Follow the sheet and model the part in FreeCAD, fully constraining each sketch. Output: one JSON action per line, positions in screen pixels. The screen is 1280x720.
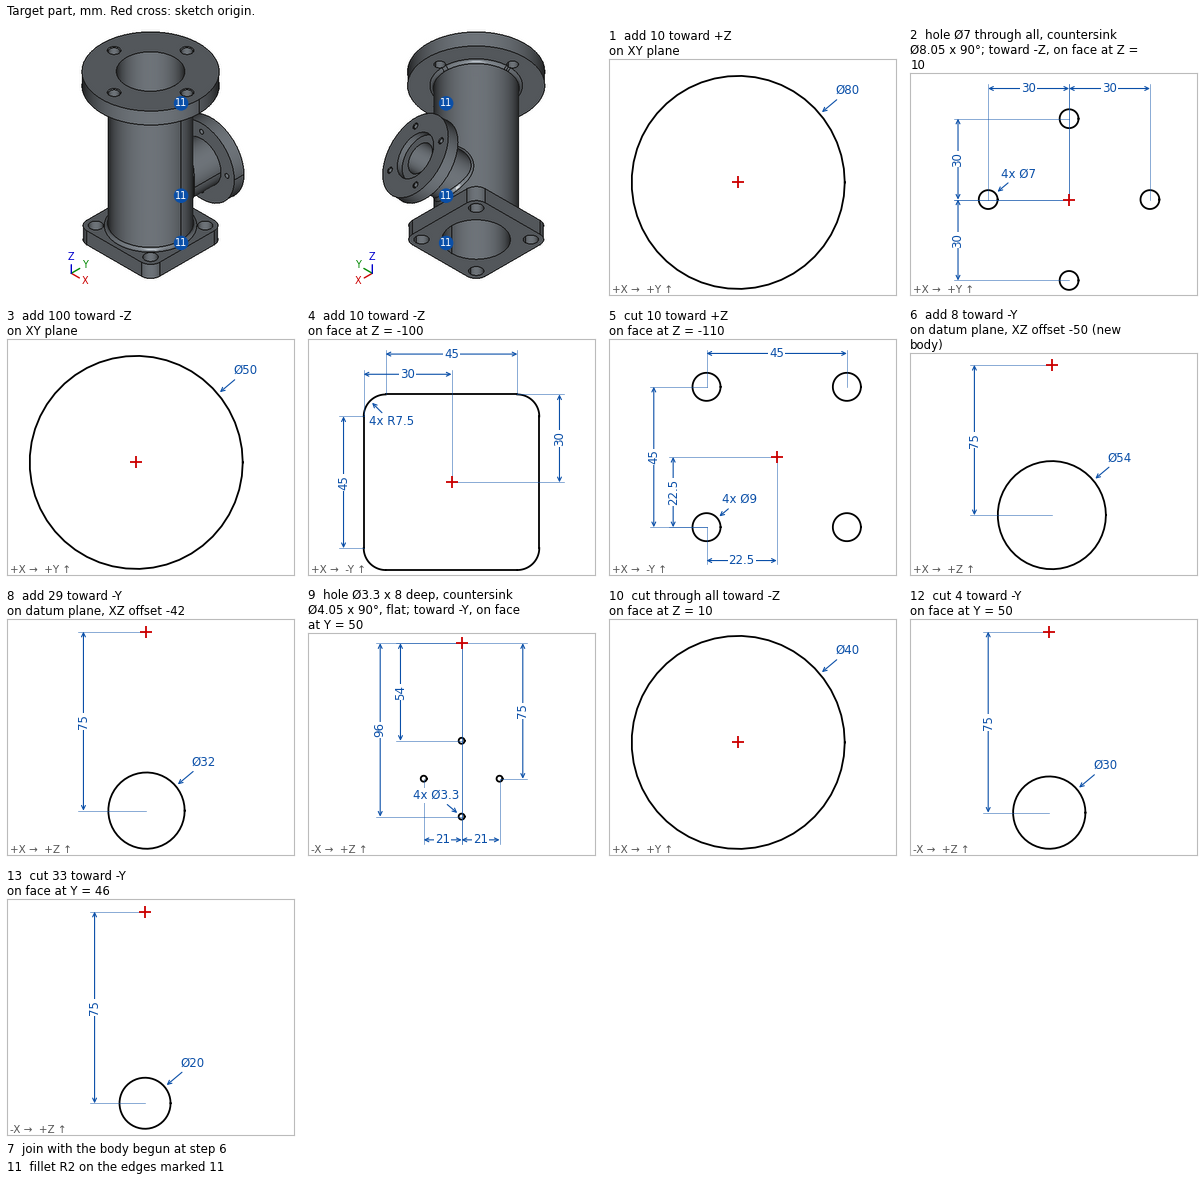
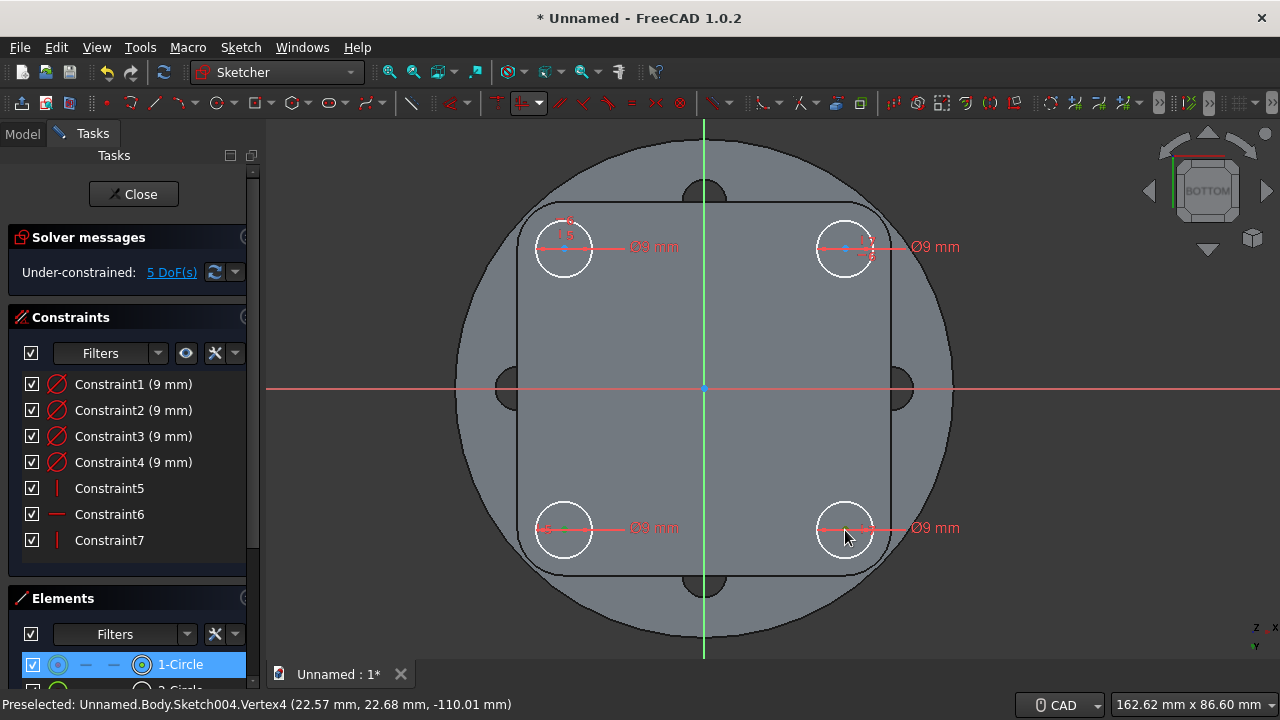
{"action": "left_click", "coordinate": [542, 104]}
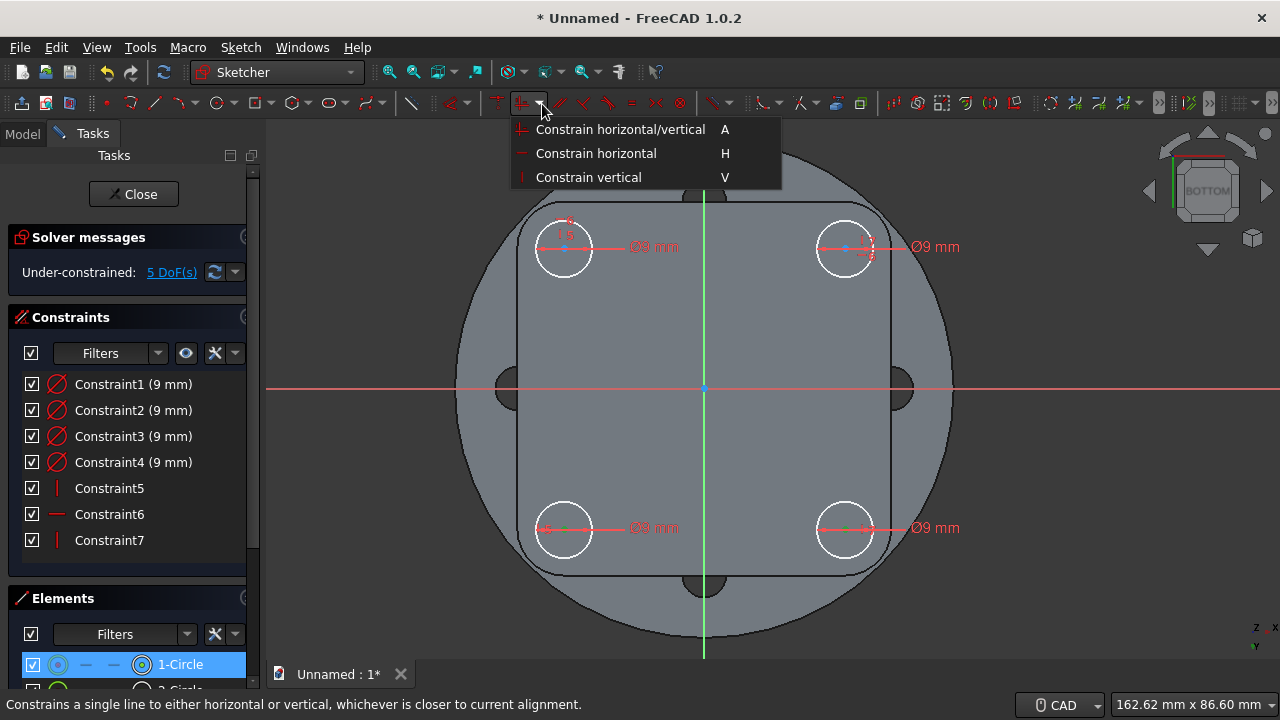
{"action": "left_click", "coordinate": [646, 153]}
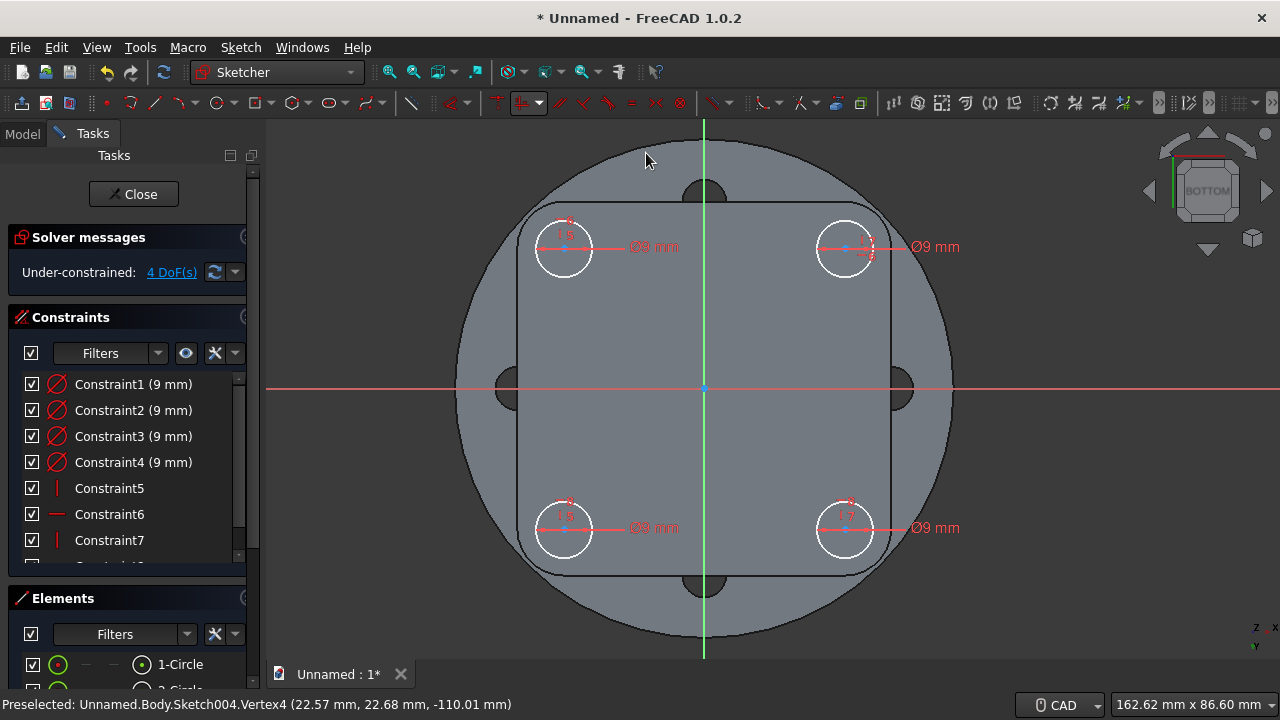
{"action": "left_click", "coordinate": [450, 104]}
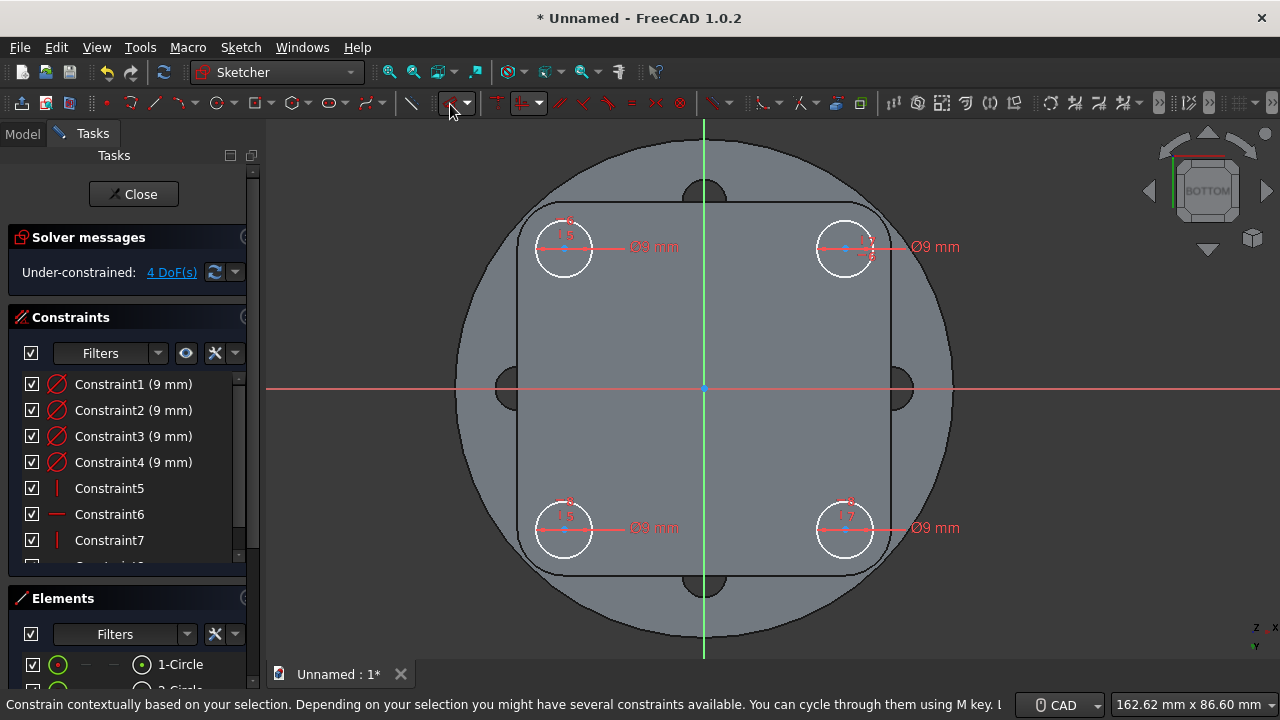
{"action": "left_click", "coordinate": [564, 530]}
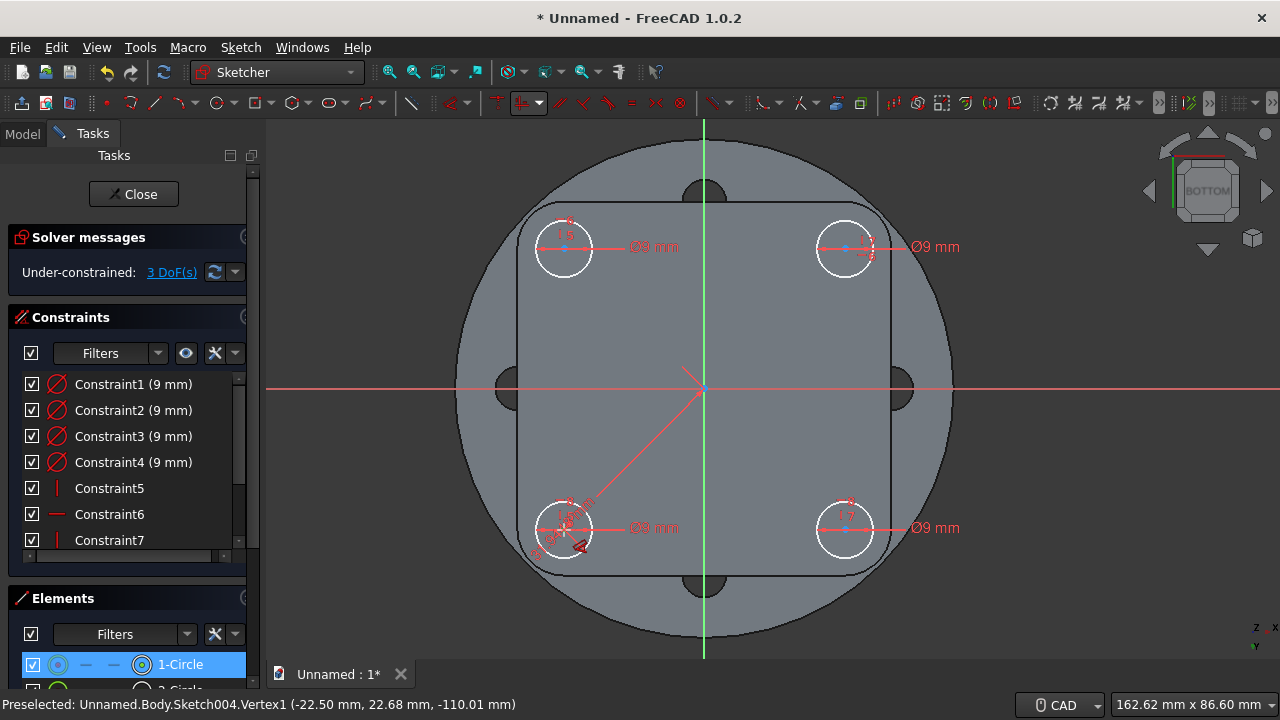
{"action": "left_click", "coordinate": [564, 249]}
{"action": "left_click", "coordinate": [530, 325]}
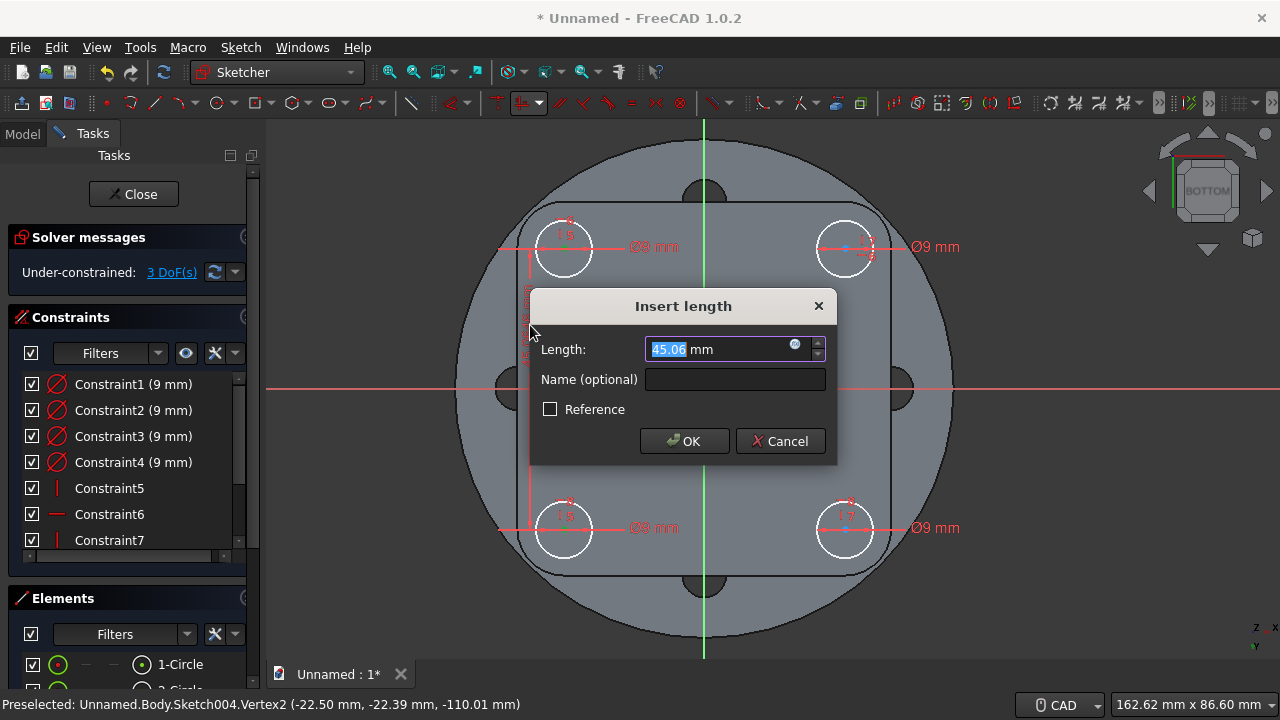
{"action": "type", "text": "45"}
{"action": "key", "text": "Return"}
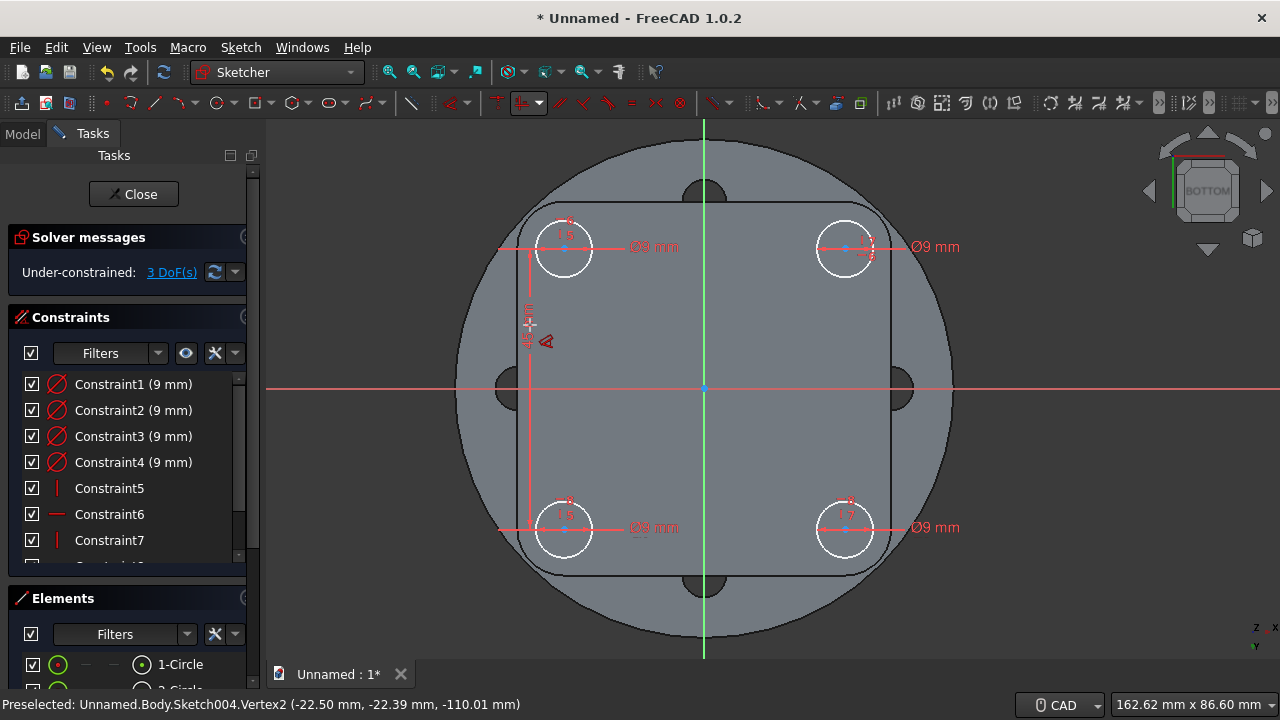
{"action": "left_click", "coordinate": [564, 249]}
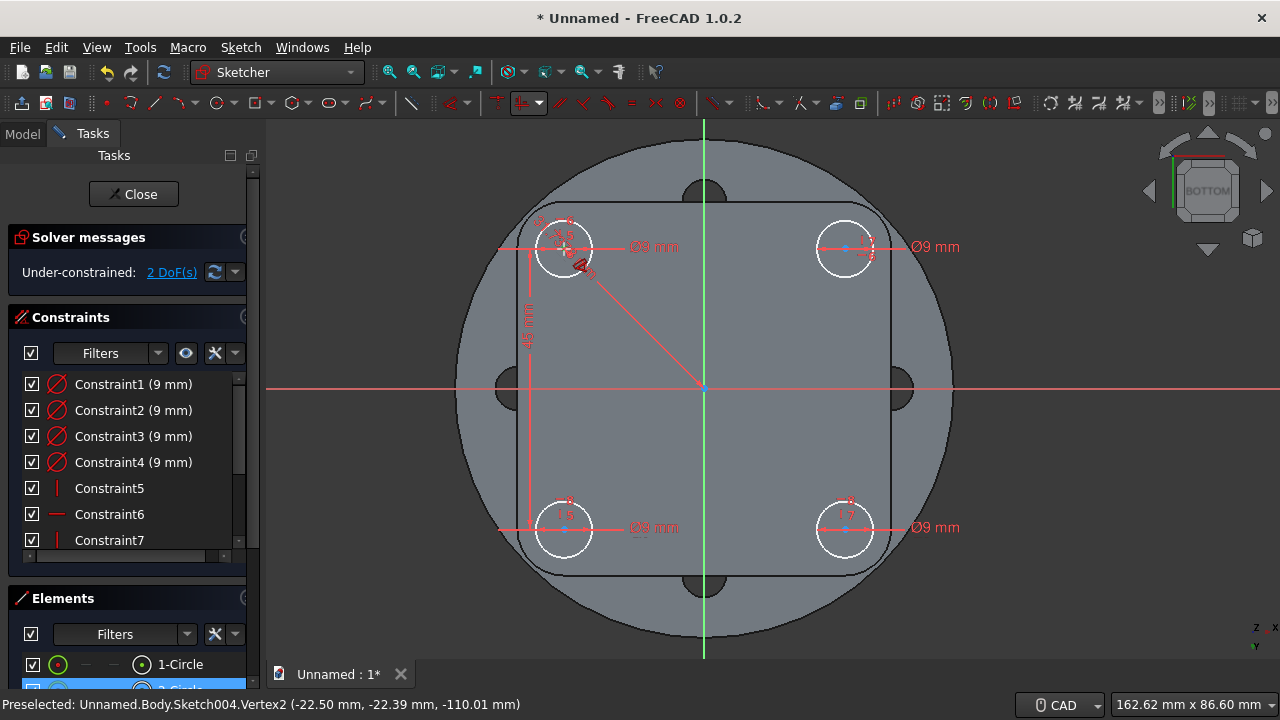
{"action": "left_click", "coordinate": [845, 249]}
{"action": "left_click", "coordinate": [640, 215]}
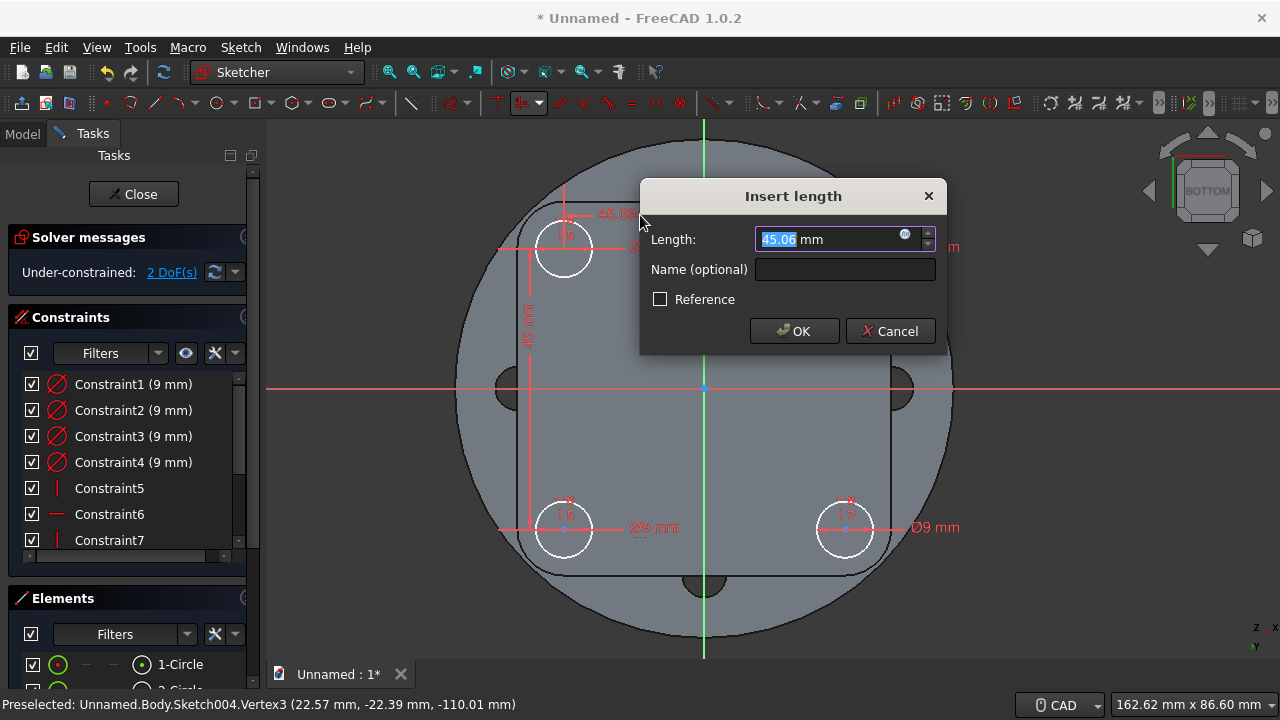
{"action": "type", "text": "45"}
{"action": "key", "text": "Return"}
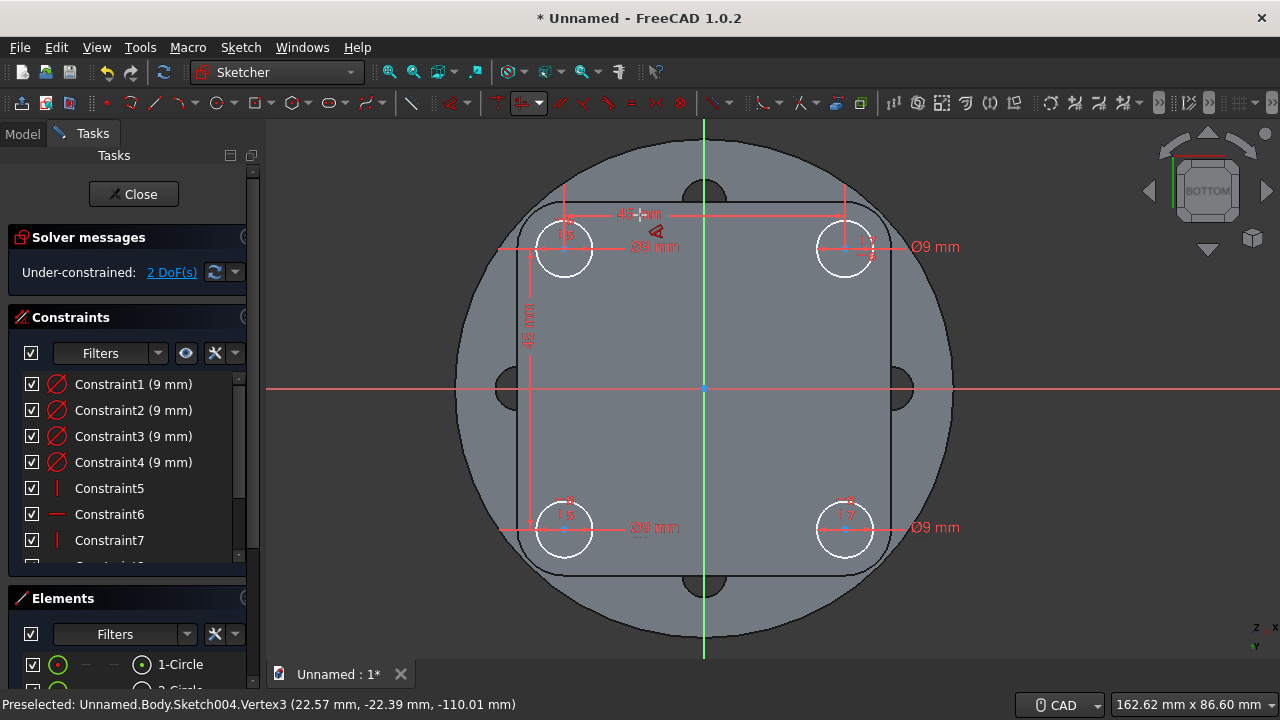
{"action": "left_click", "coordinate": [564, 530]}
{"action": "left_click", "coordinate": [634, 564]}